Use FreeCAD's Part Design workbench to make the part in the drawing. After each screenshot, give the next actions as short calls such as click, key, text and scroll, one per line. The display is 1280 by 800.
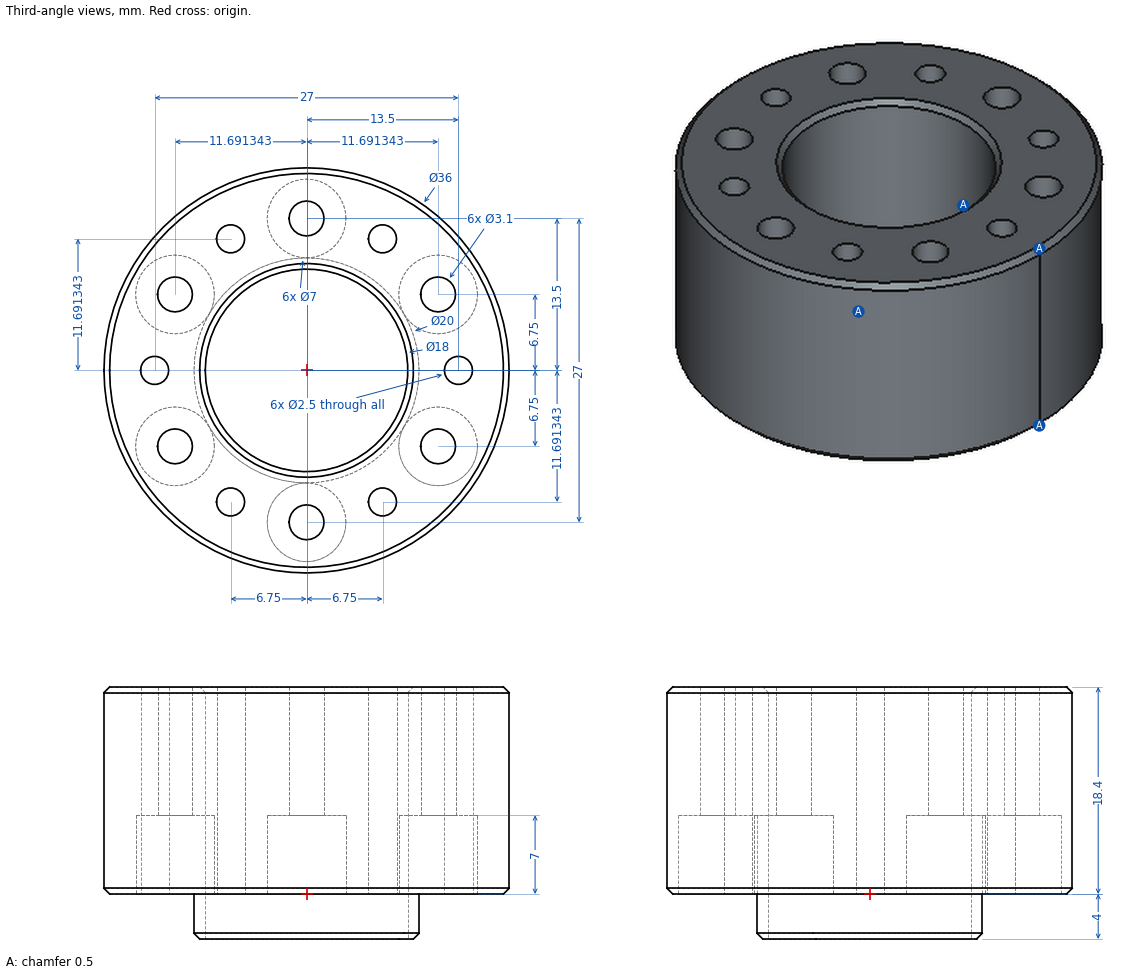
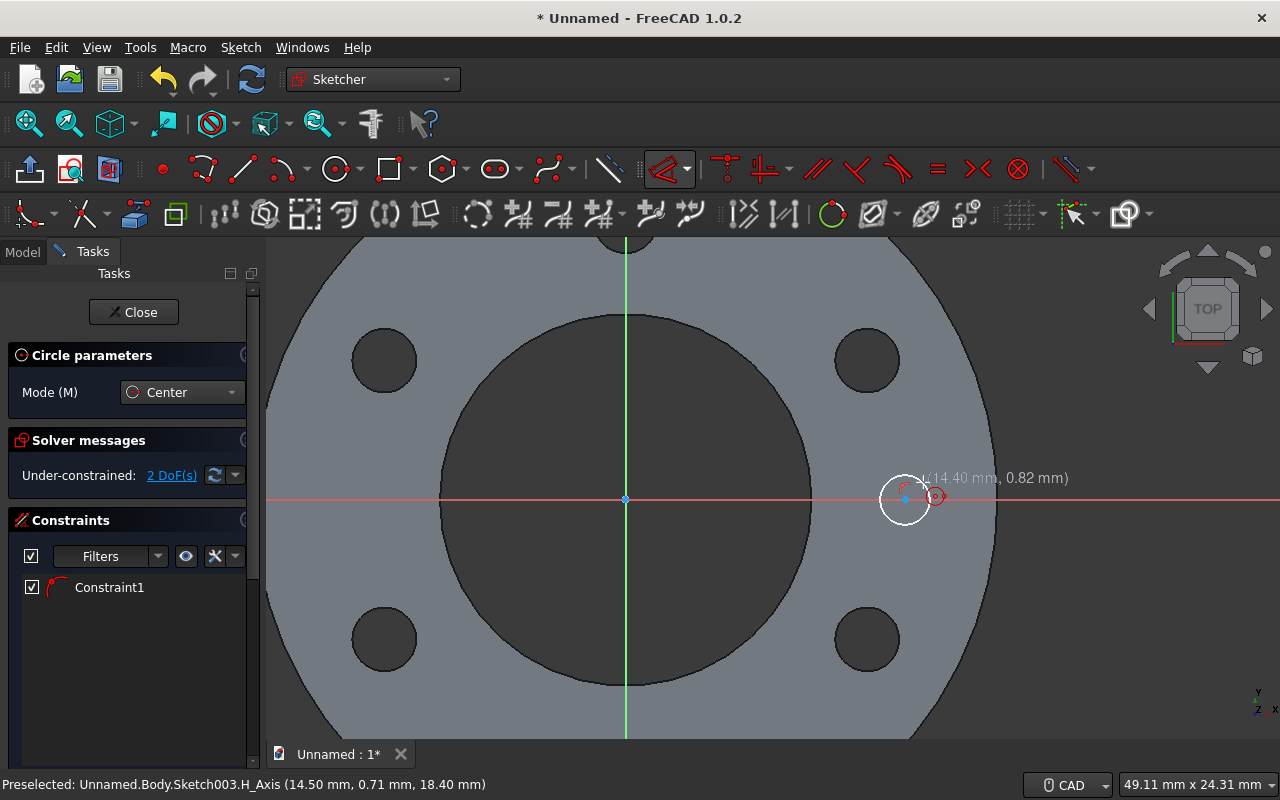
scroll(800, 473, down, 3)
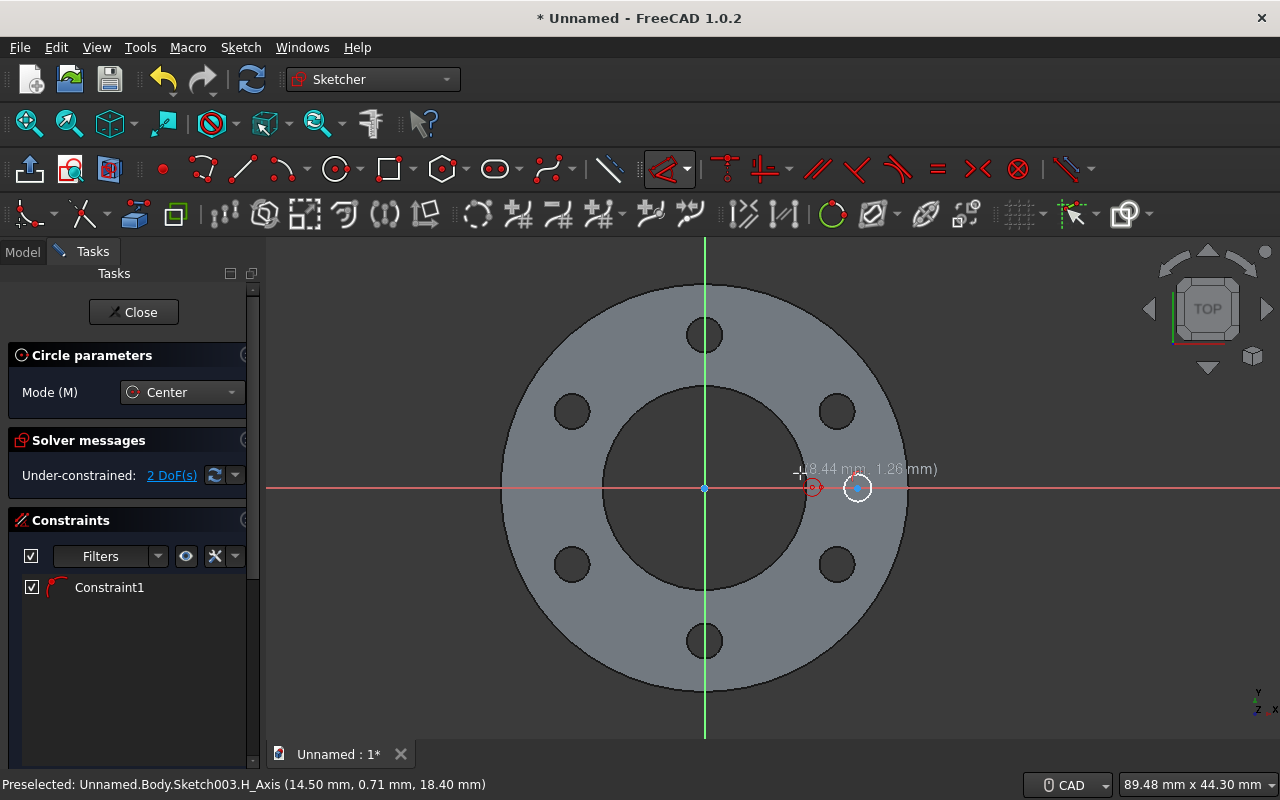
scroll(781, 621, up, 3)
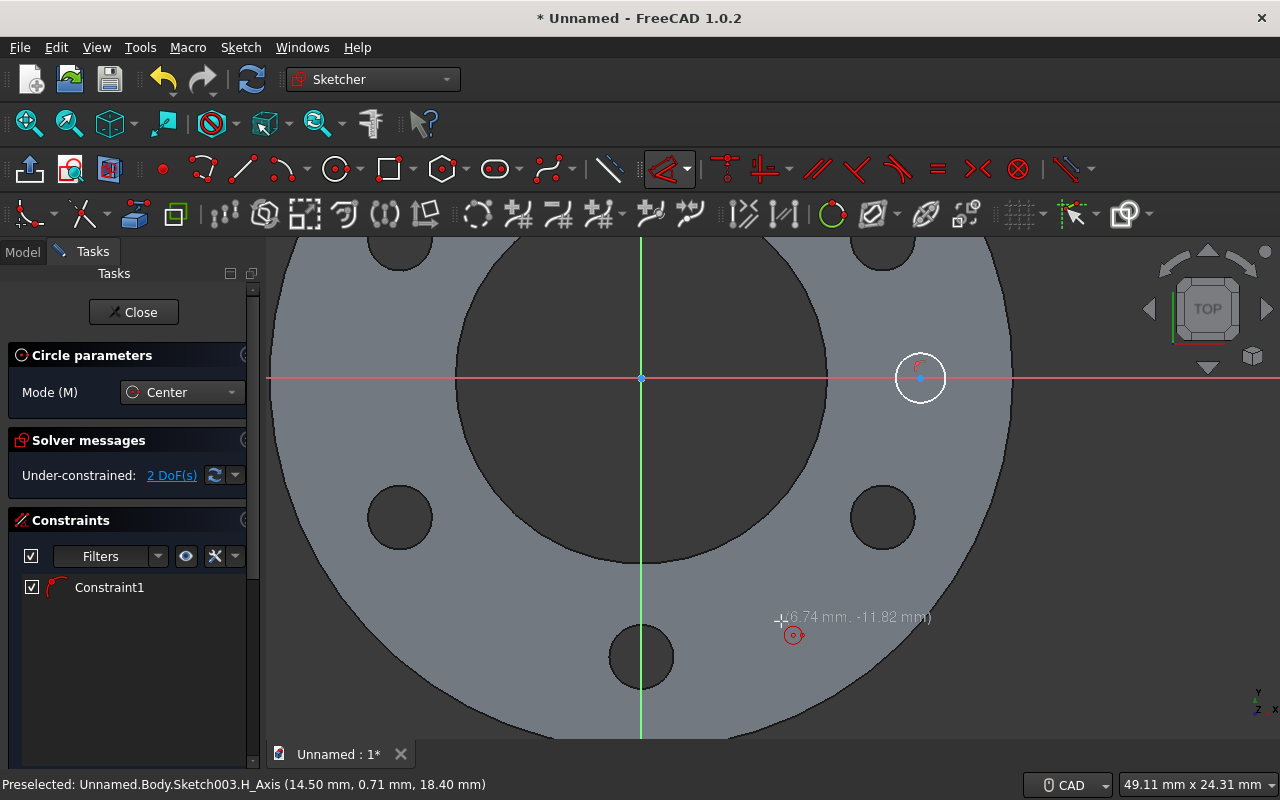
click(781, 619)
click(799, 601)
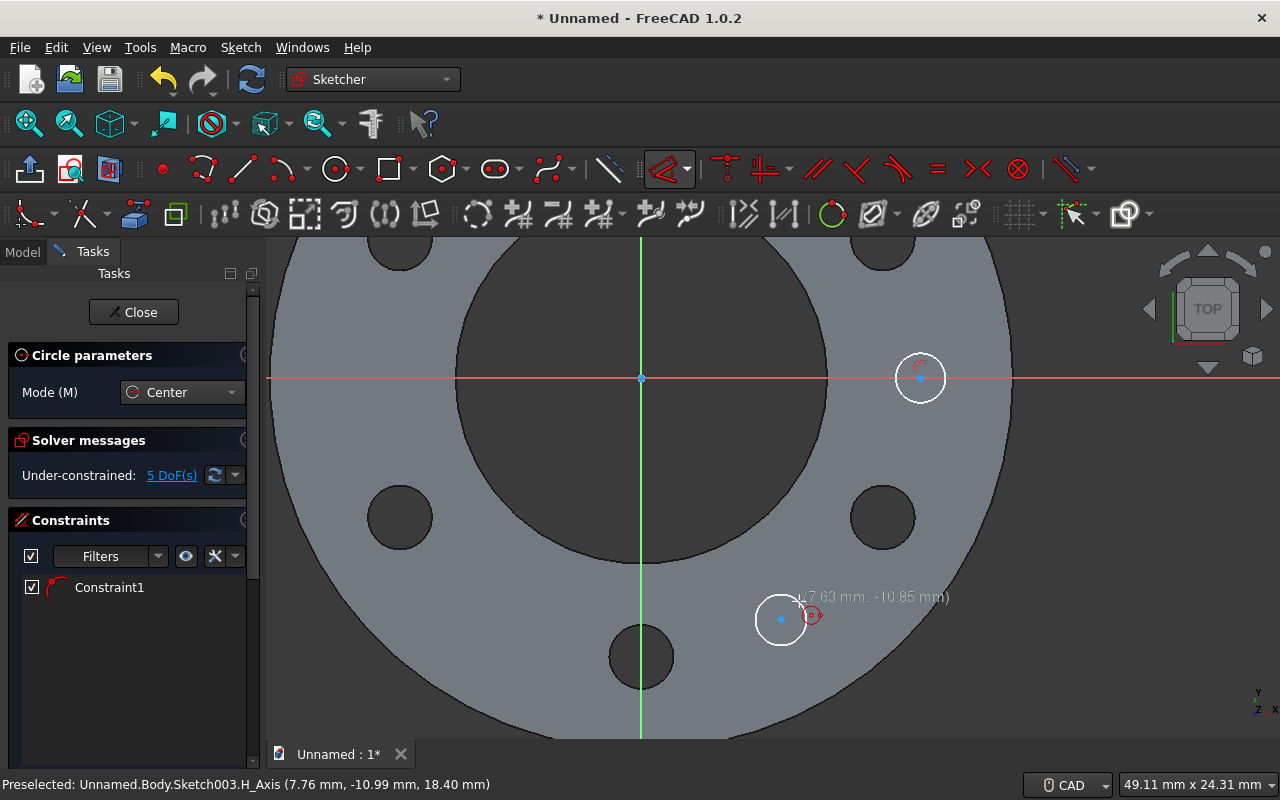
click(502, 619)
click(520, 601)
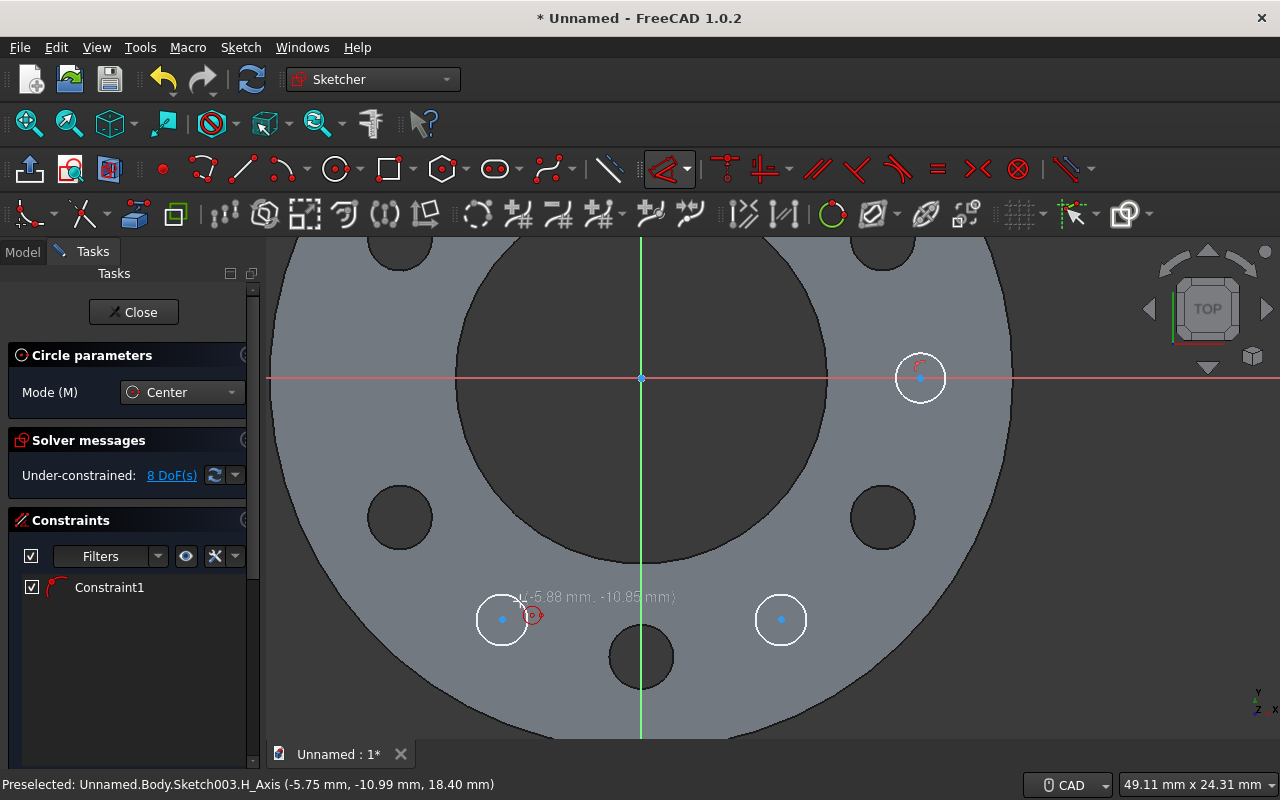
click(363, 378)
click(381, 360)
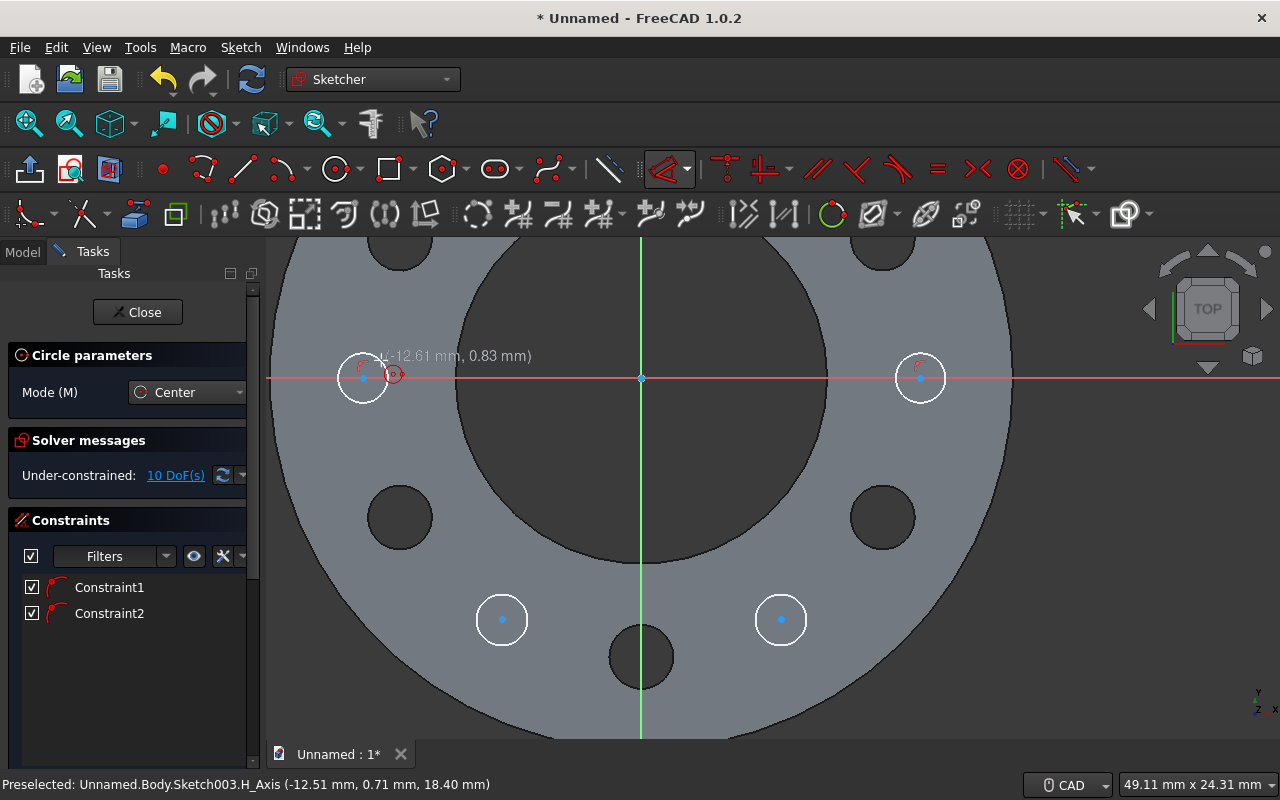
scroll(781, 622, down, 3)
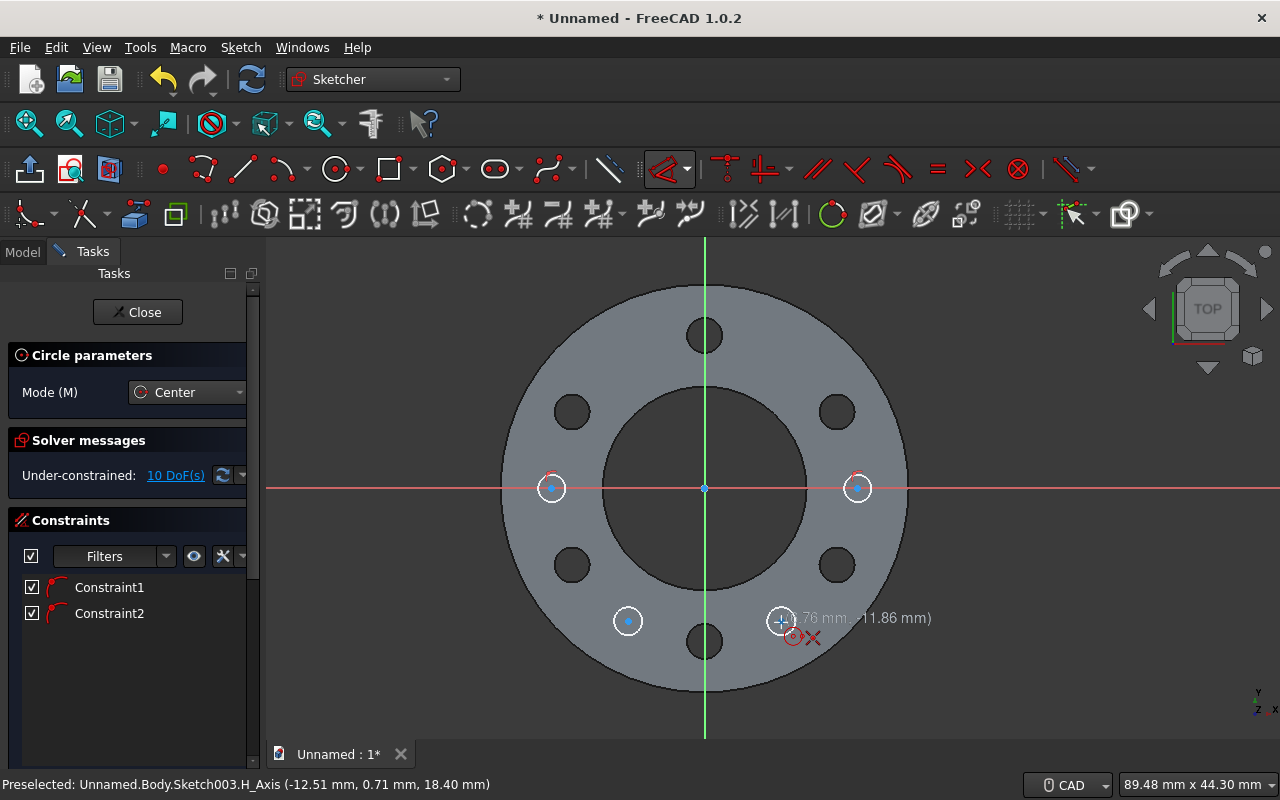
scroll(628, 356, up, 3)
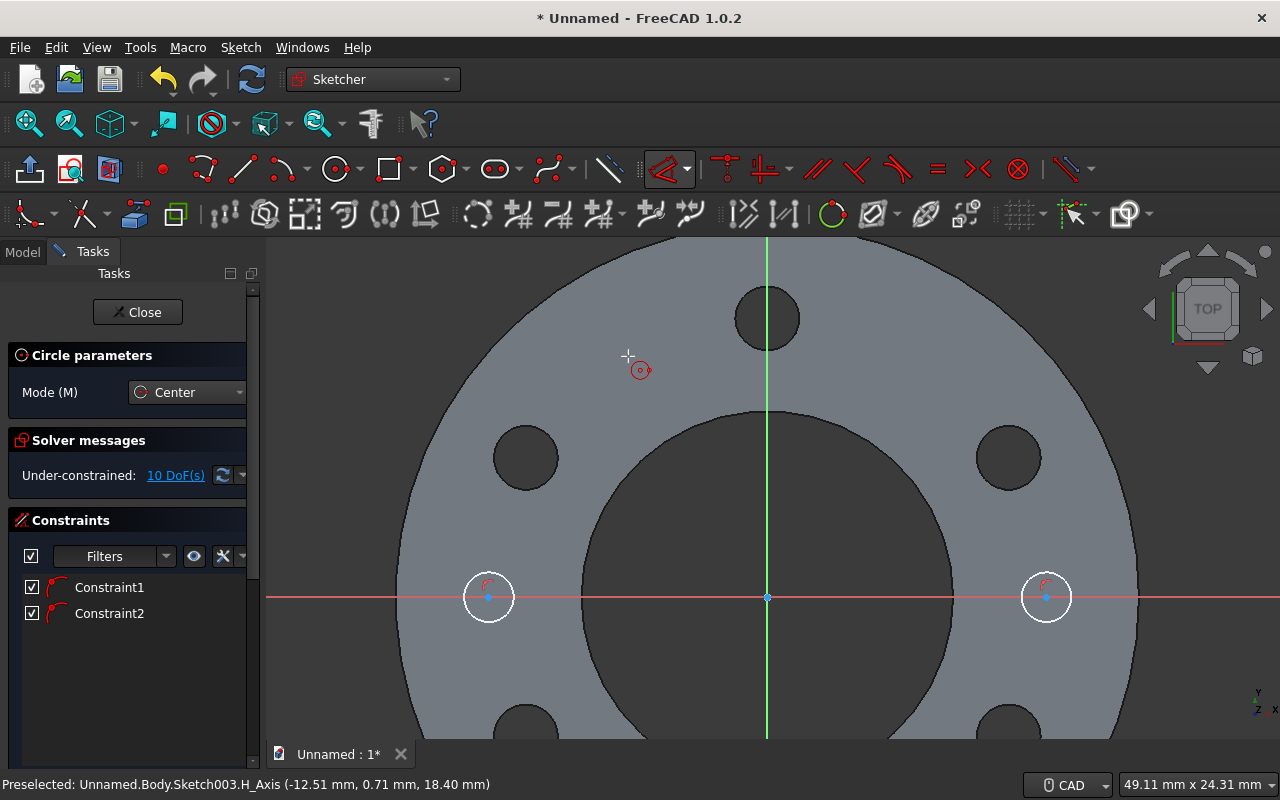
click(628, 356)
click(646, 337)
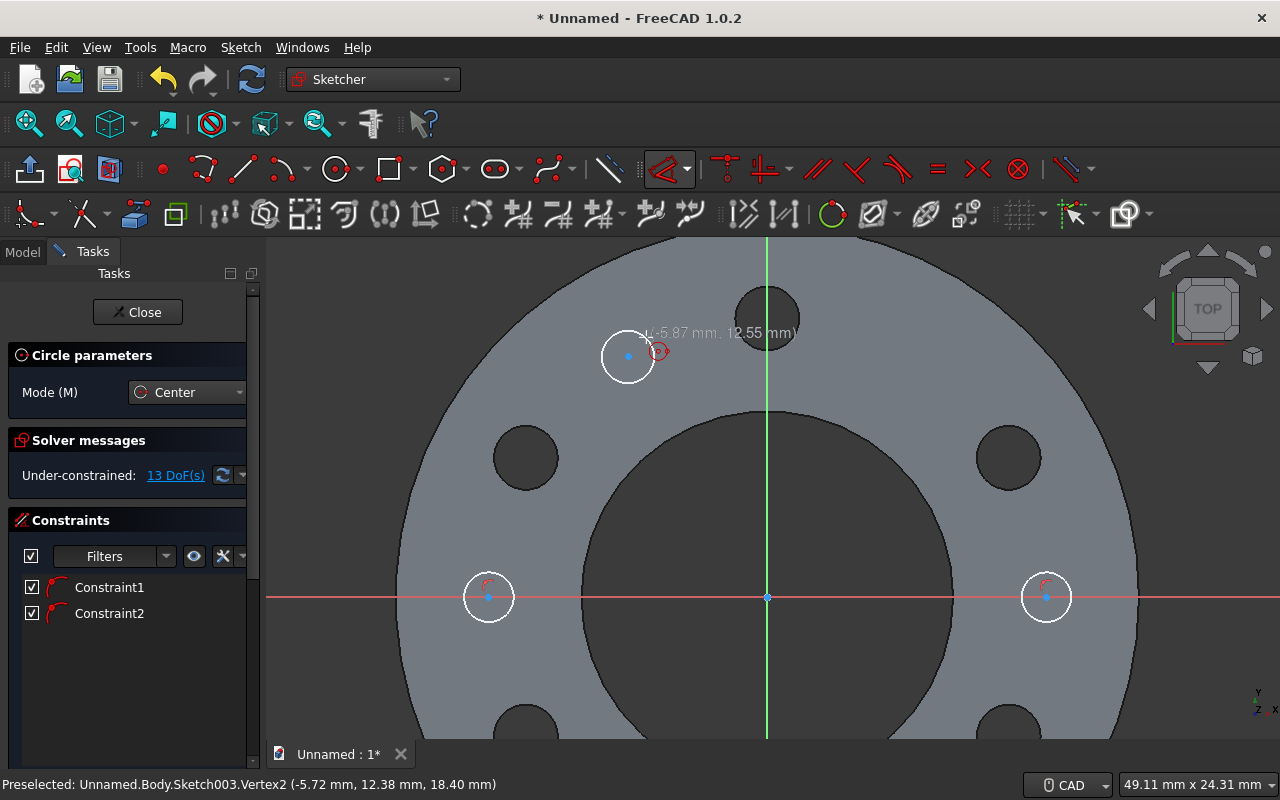
click(907, 356)
click(925, 337)
key(Escape)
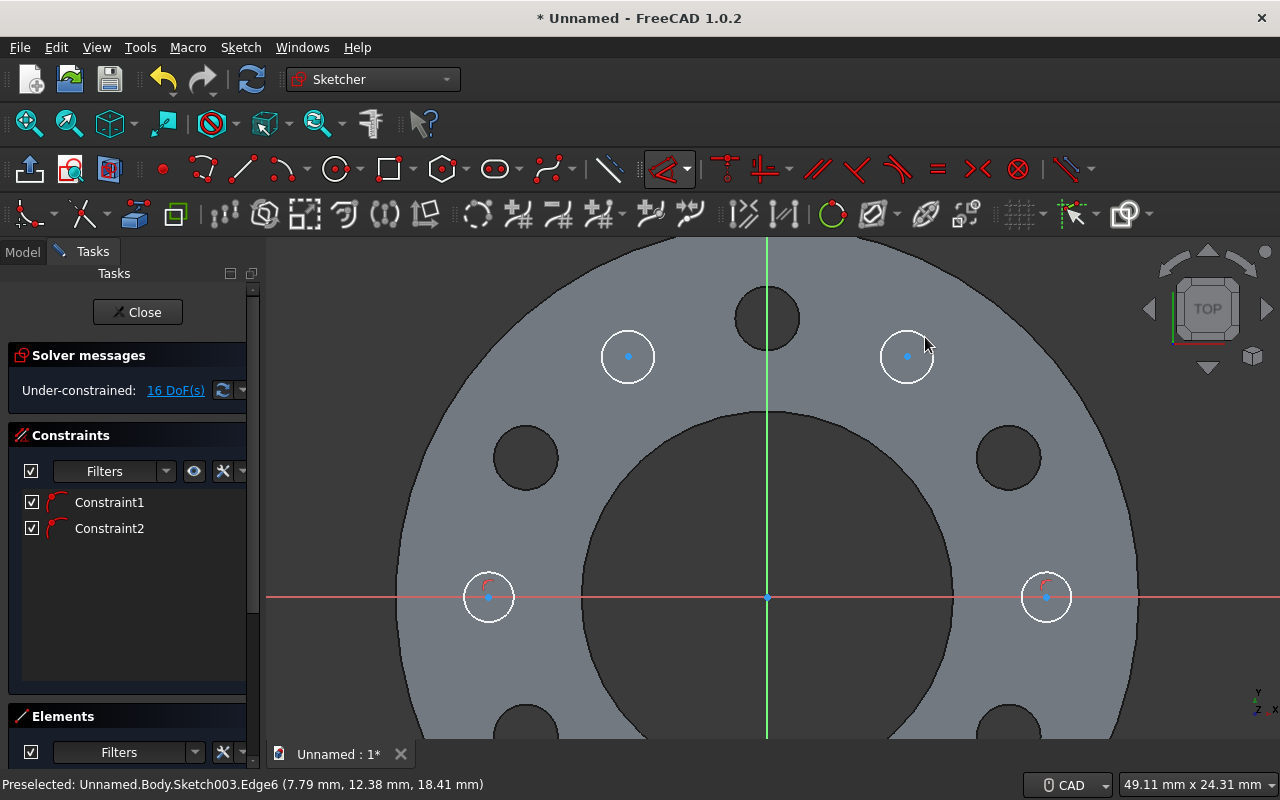
click(1064, 580)